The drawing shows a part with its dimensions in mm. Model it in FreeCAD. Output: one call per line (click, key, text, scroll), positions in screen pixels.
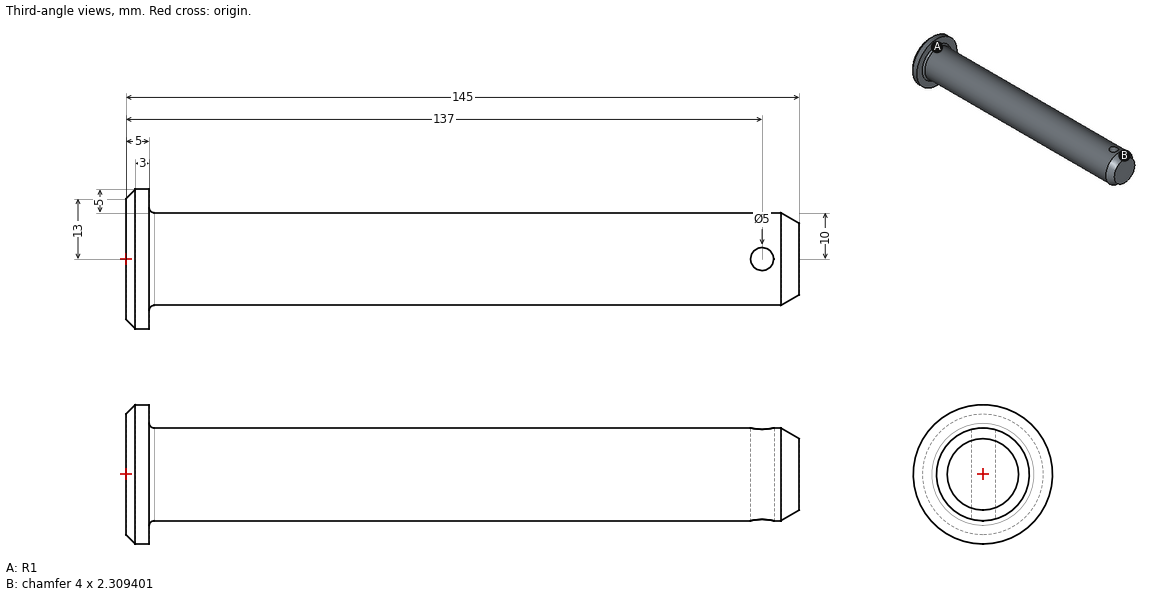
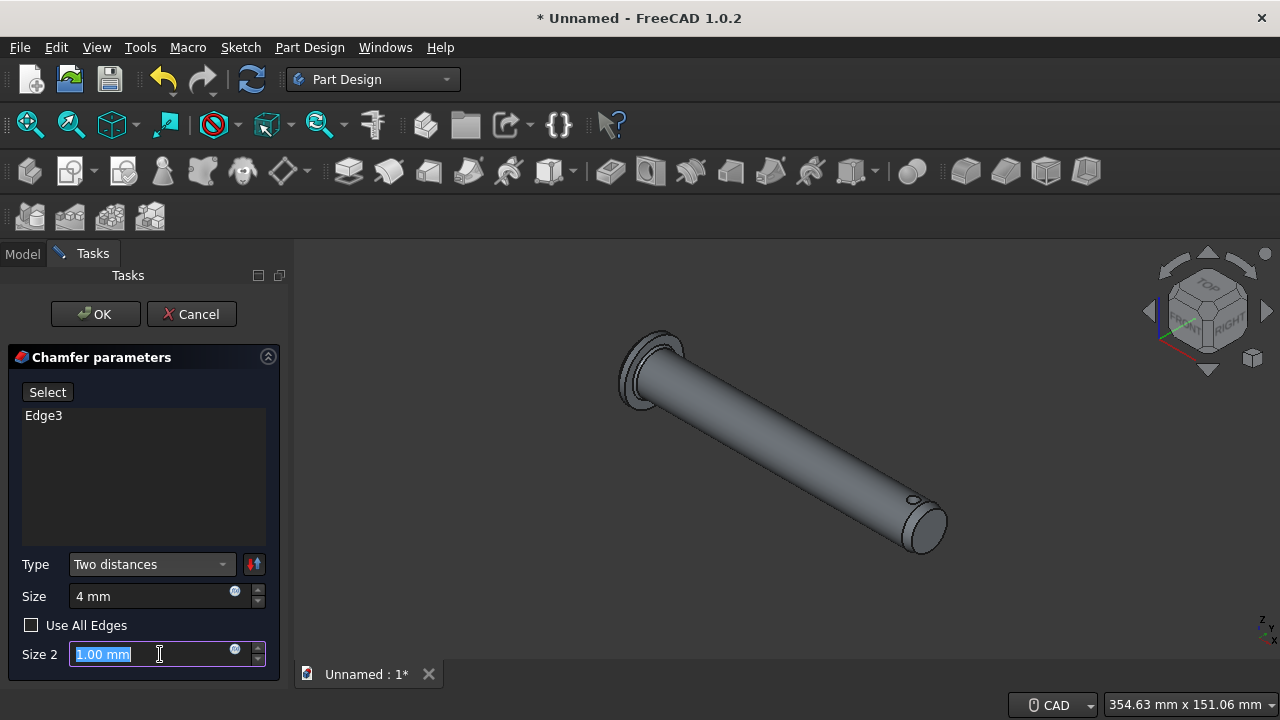
text(2.309401)
key(Tab)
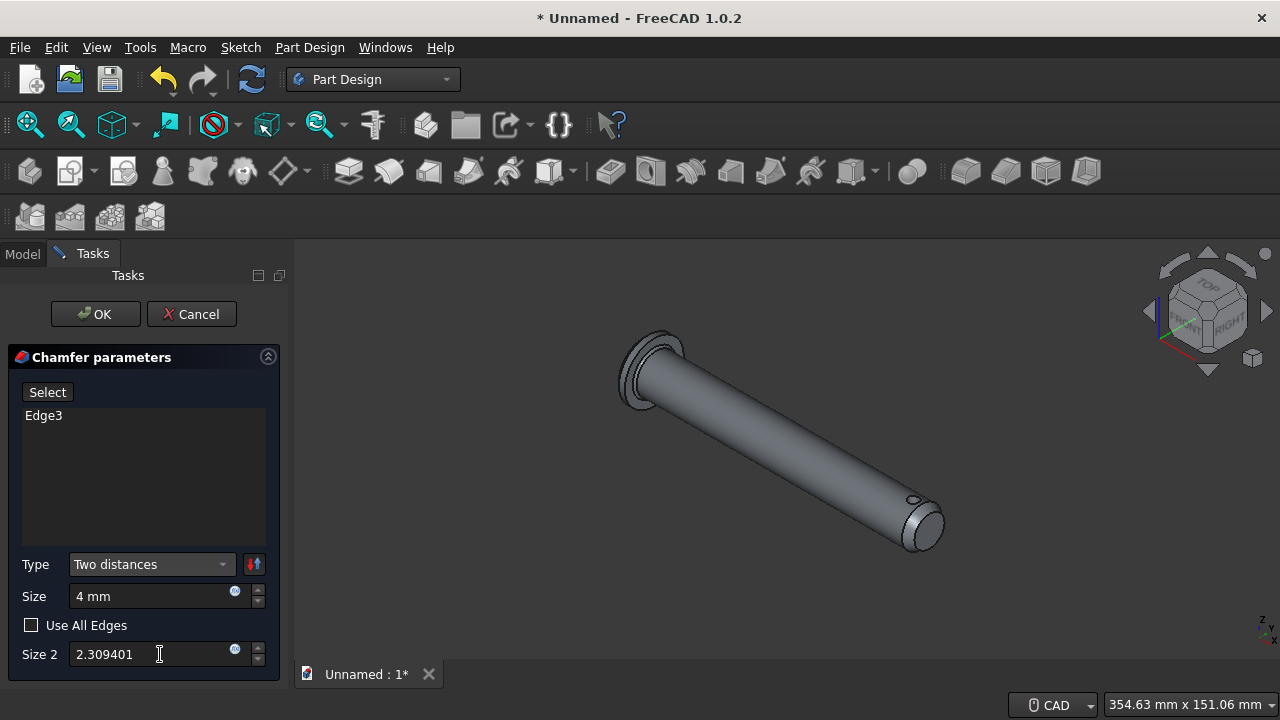
click(96, 314)